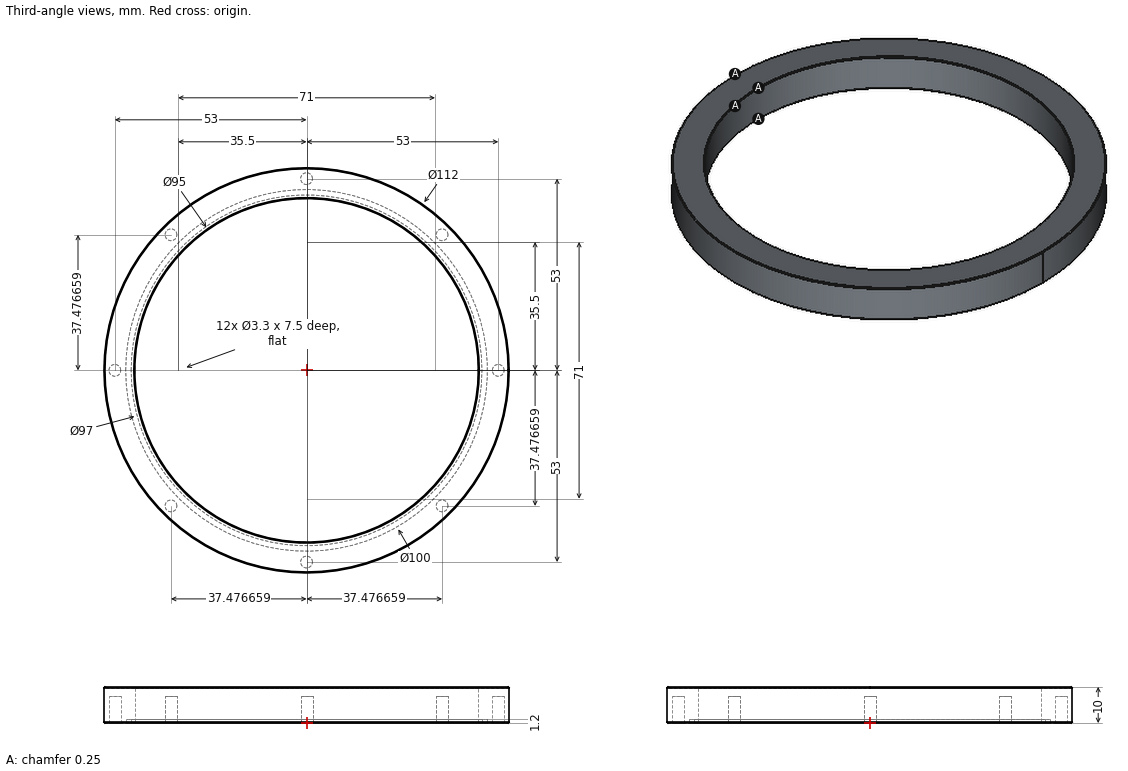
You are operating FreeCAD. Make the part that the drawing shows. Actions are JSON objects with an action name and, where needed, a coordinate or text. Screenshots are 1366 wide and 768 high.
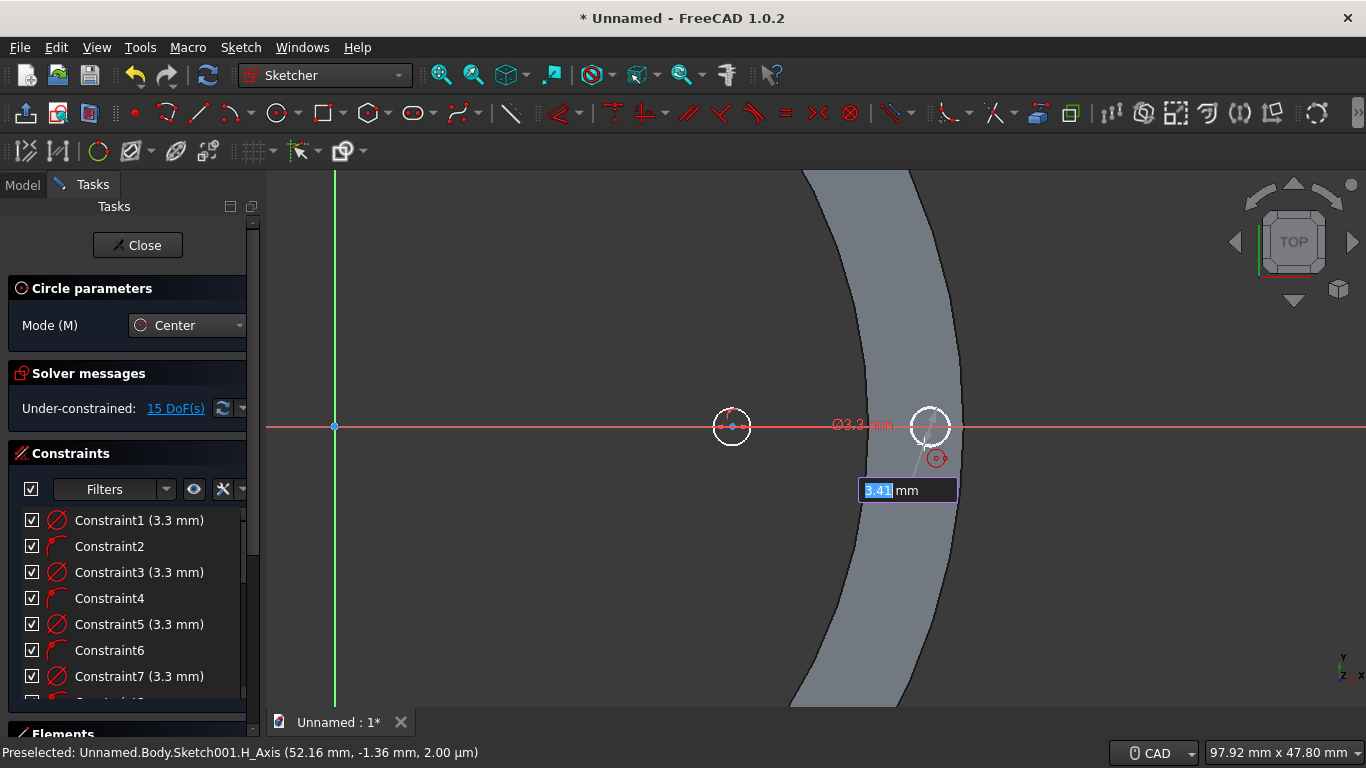
{"action": "type", "text": "3.3"}
{"action": "key", "text": "Return"}
{"action": "key", "text": "Escape"}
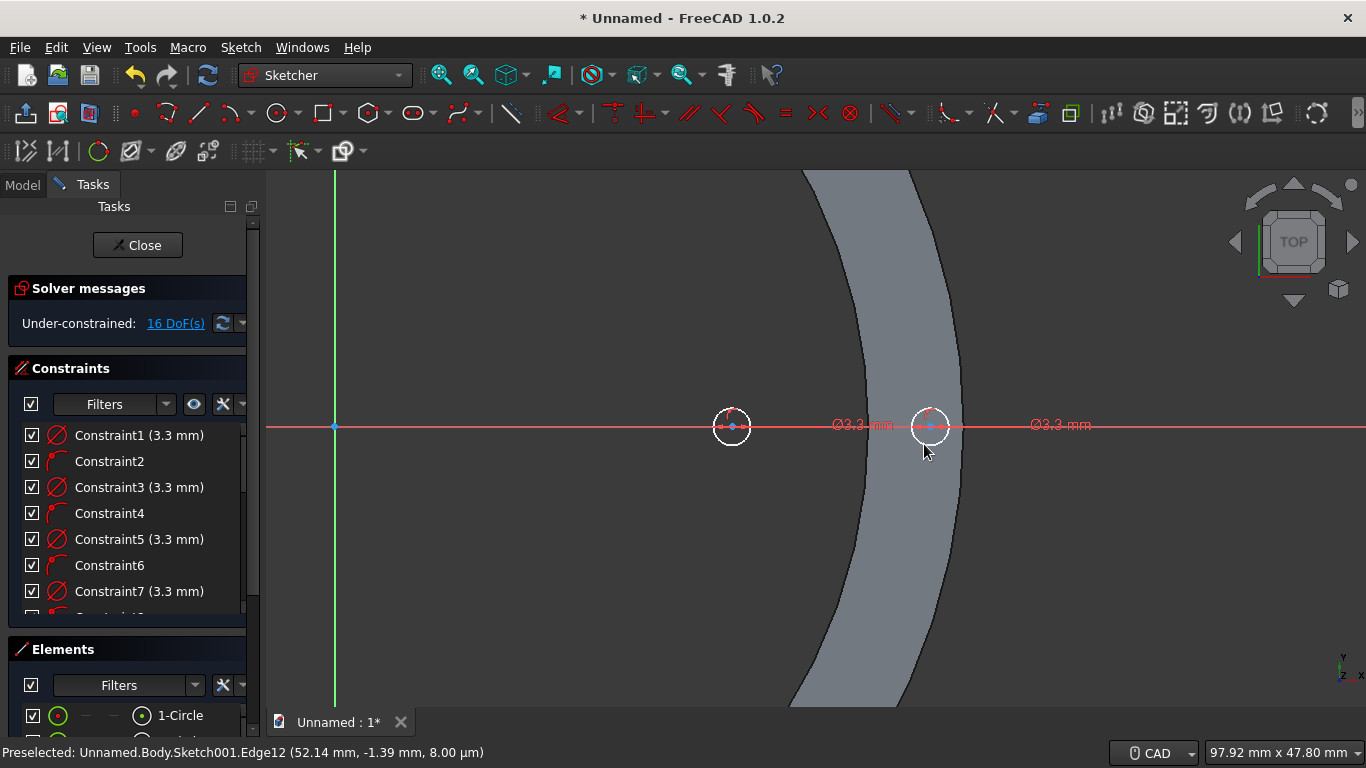
{"action": "left_click", "coordinate": [558, 114]}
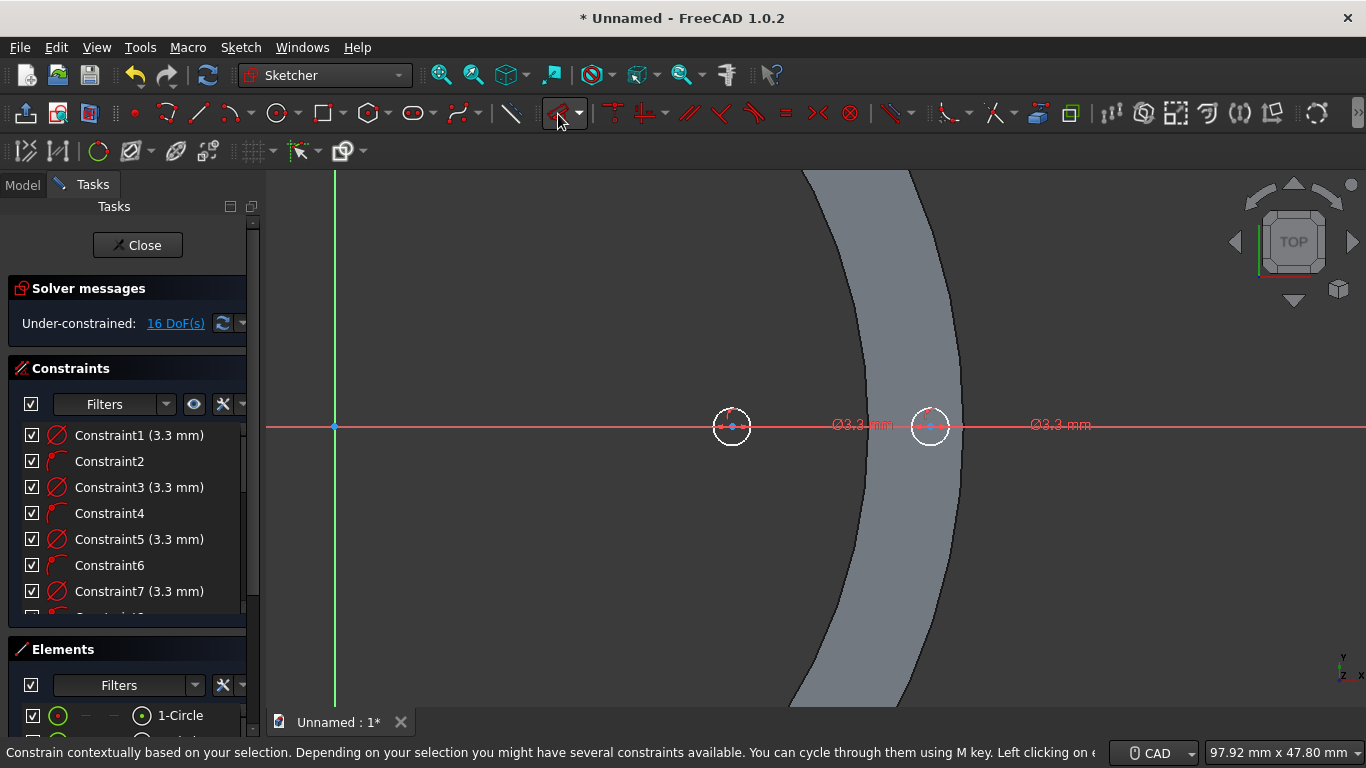
{"action": "scroll", "coordinate": [925, 444], "scroll_direction": "down", "scroll_amount": 6}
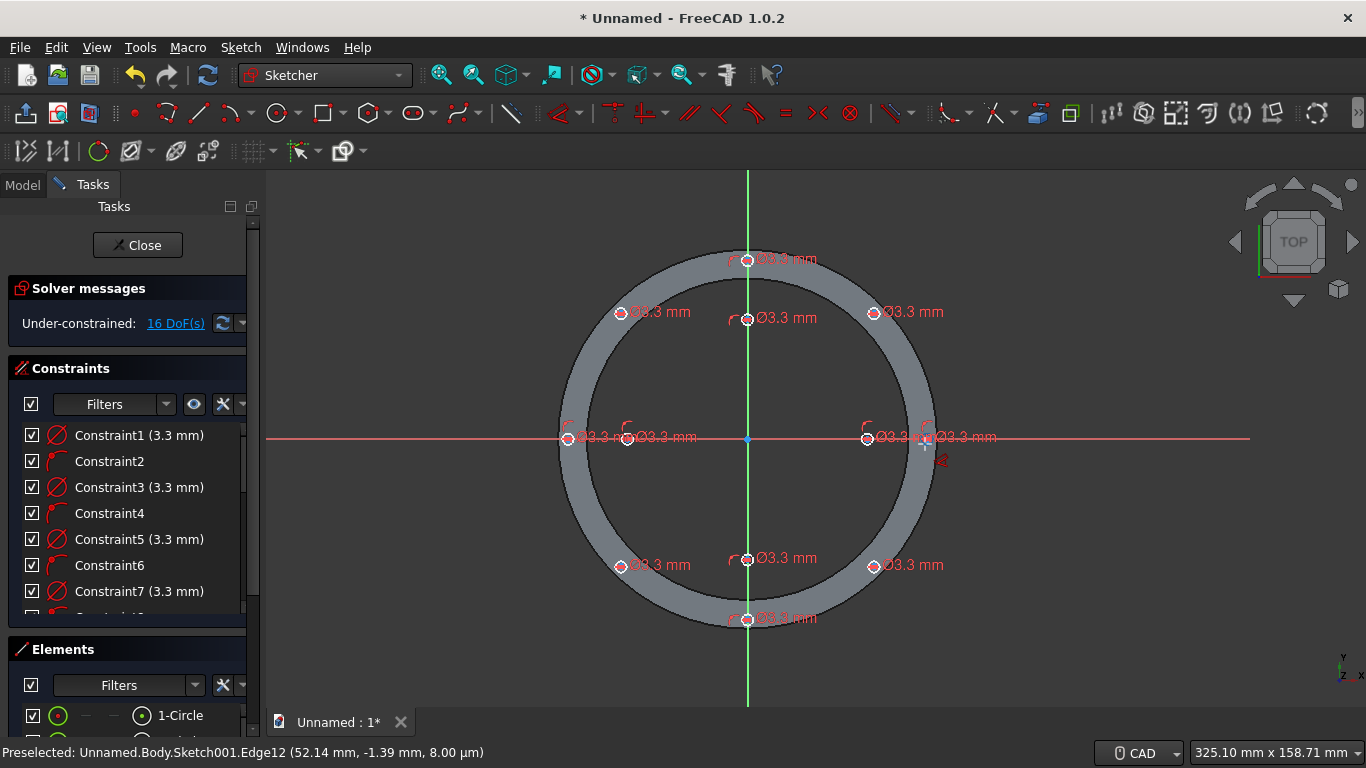
{"action": "left_click", "coordinate": [748, 261]}
{"action": "left_click", "coordinate": [782, 350]}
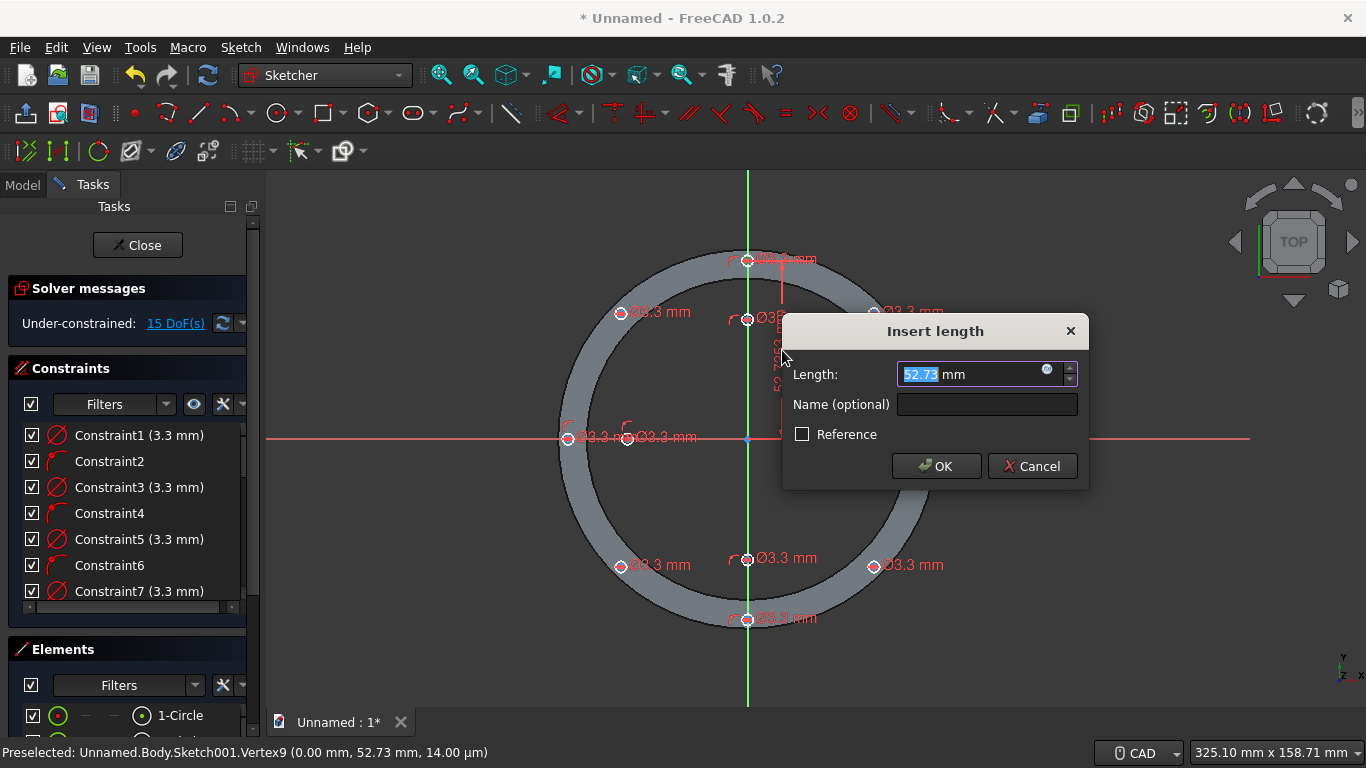
{"action": "type", "text": "53"}
{"action": "key", "text": "Return"}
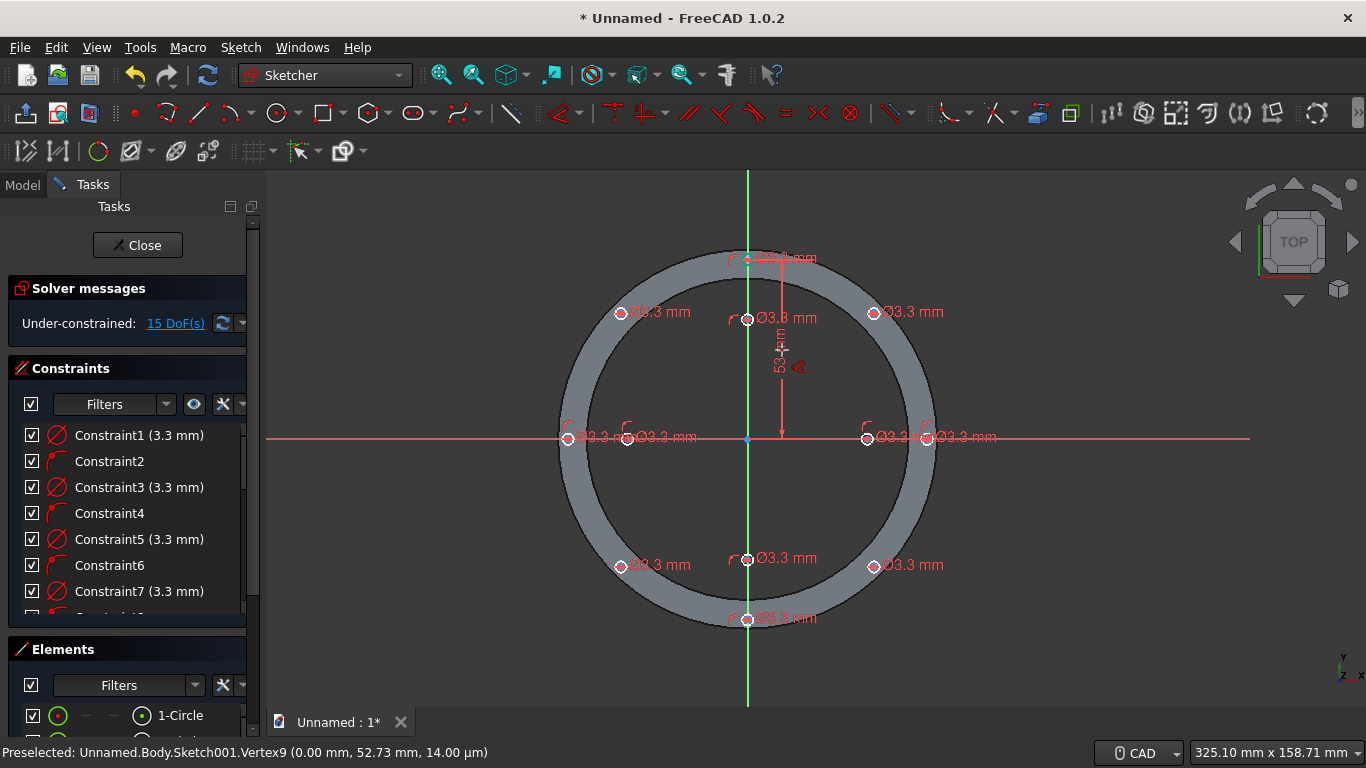
{"action": "left_click", "coordinate": [568, 439]}
{"action": "left_click", "coordinate": [658, 473]}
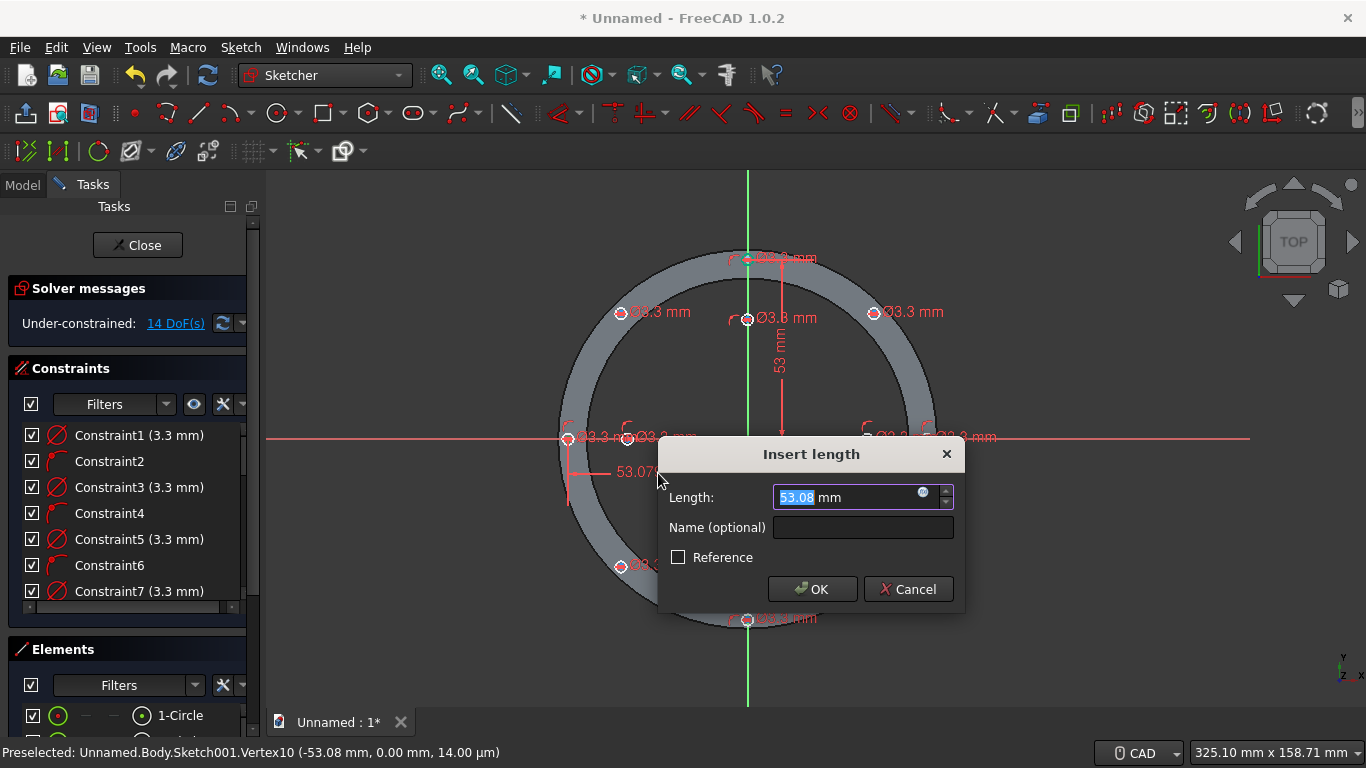
{"action": "type", "text": "53"}
{"action": "key", "text": "Return"}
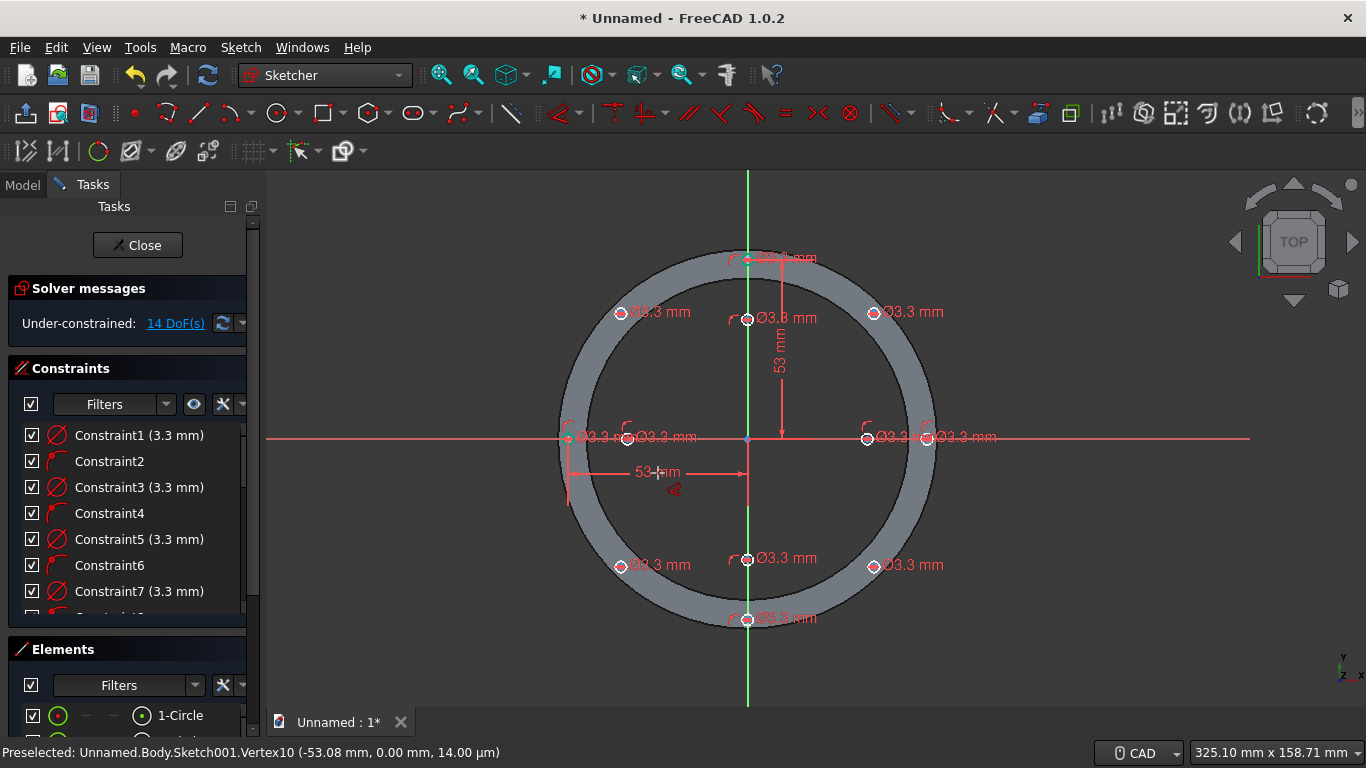
{"action": "left_click", "coordinate": [748, 620]}
{"action": "left_click", "coordinate": [782, 530]}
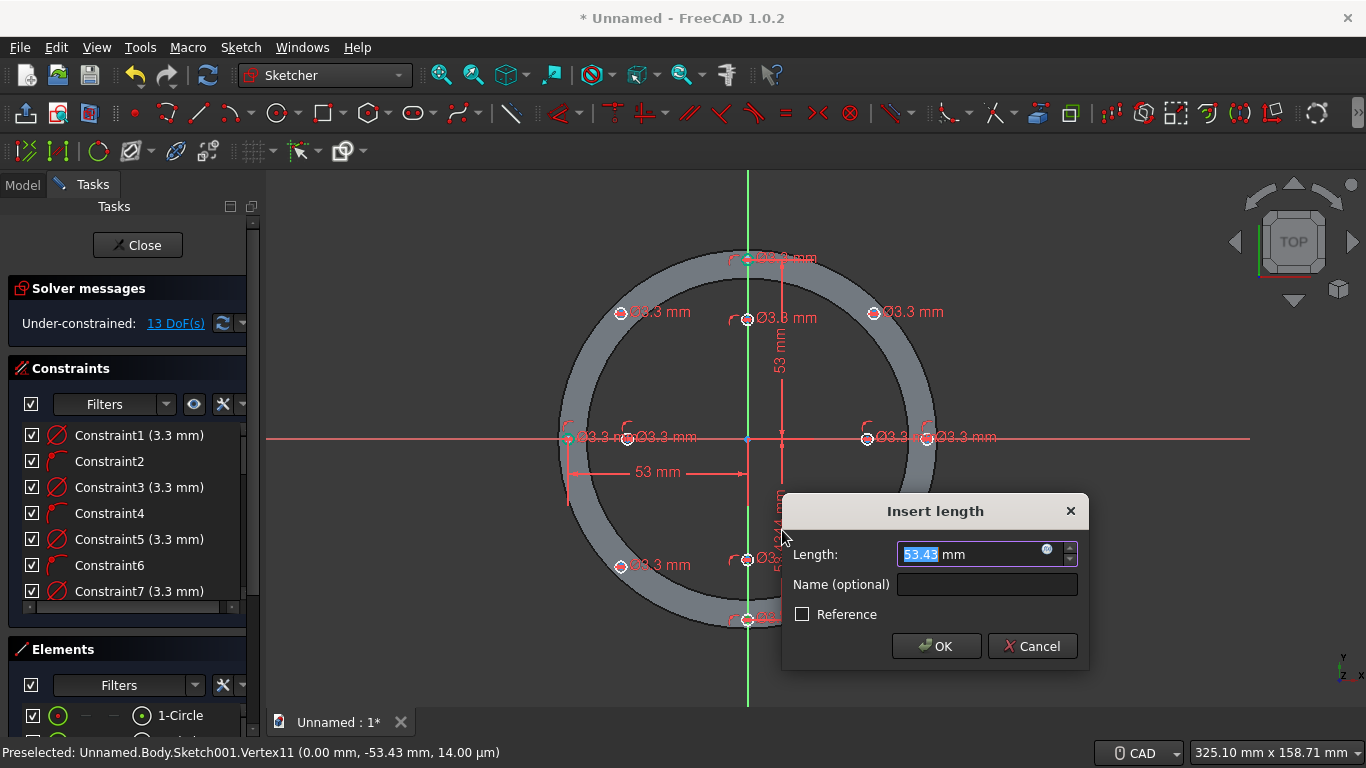
{"action": "type", "text": "53"}
{"action": "key", "text": "Return"}